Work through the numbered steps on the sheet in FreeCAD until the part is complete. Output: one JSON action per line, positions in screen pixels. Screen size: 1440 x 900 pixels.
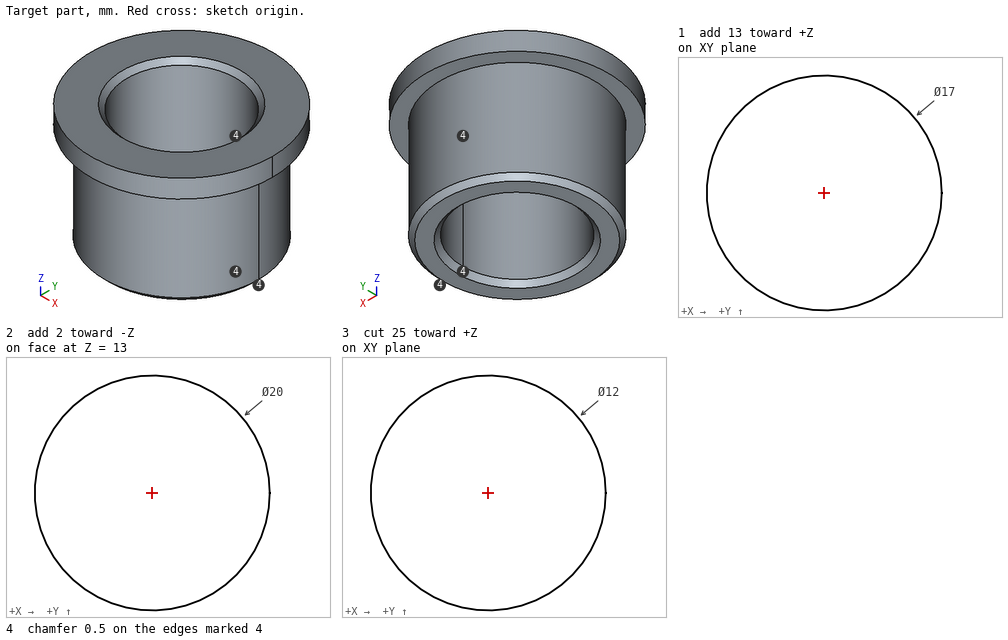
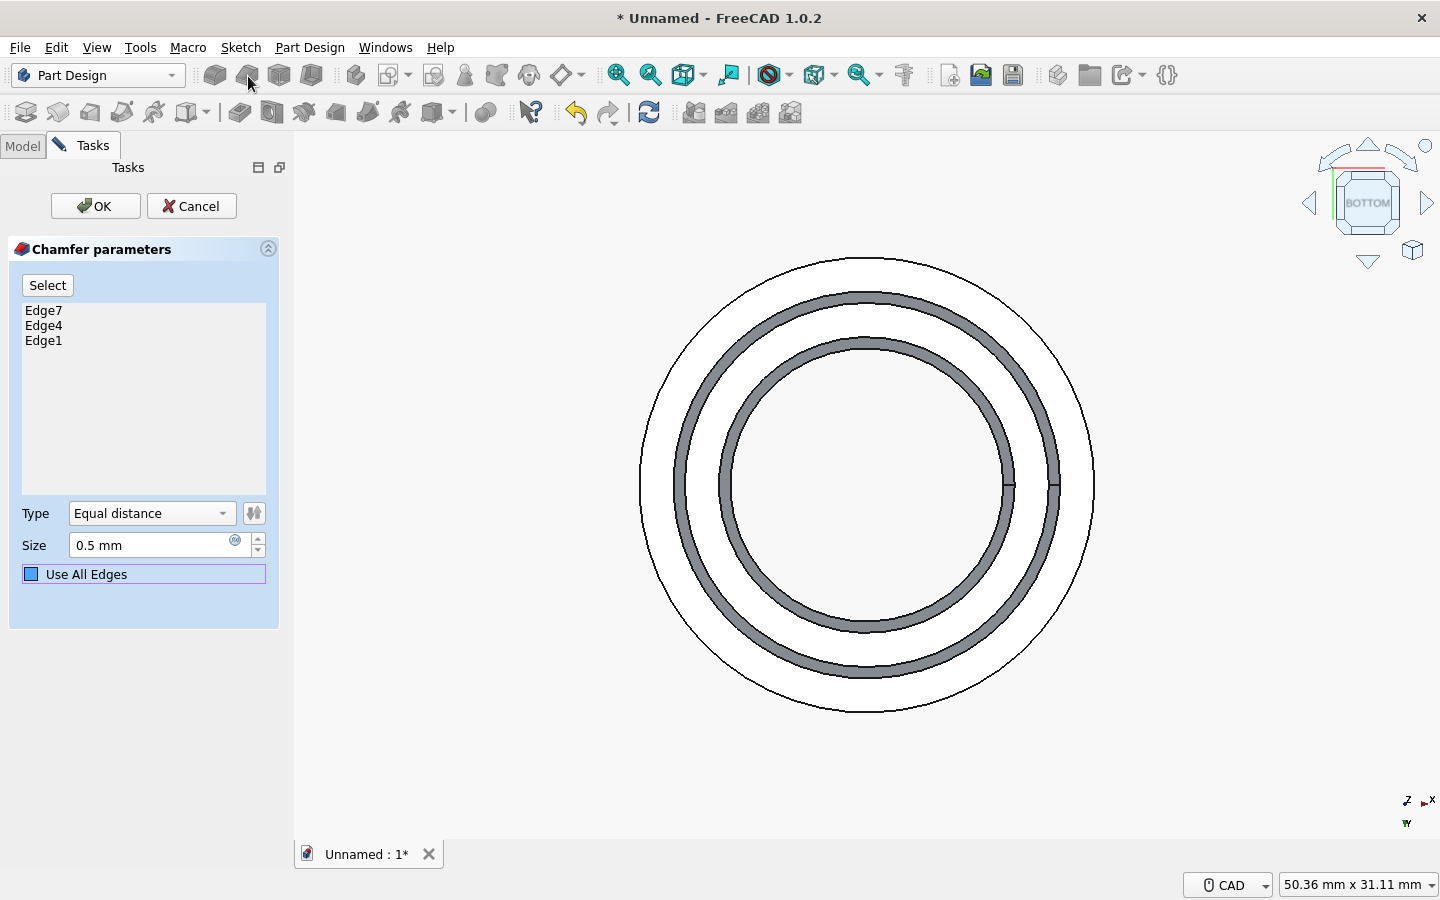
{"action": "left_click", "coordinate": [96, 206]}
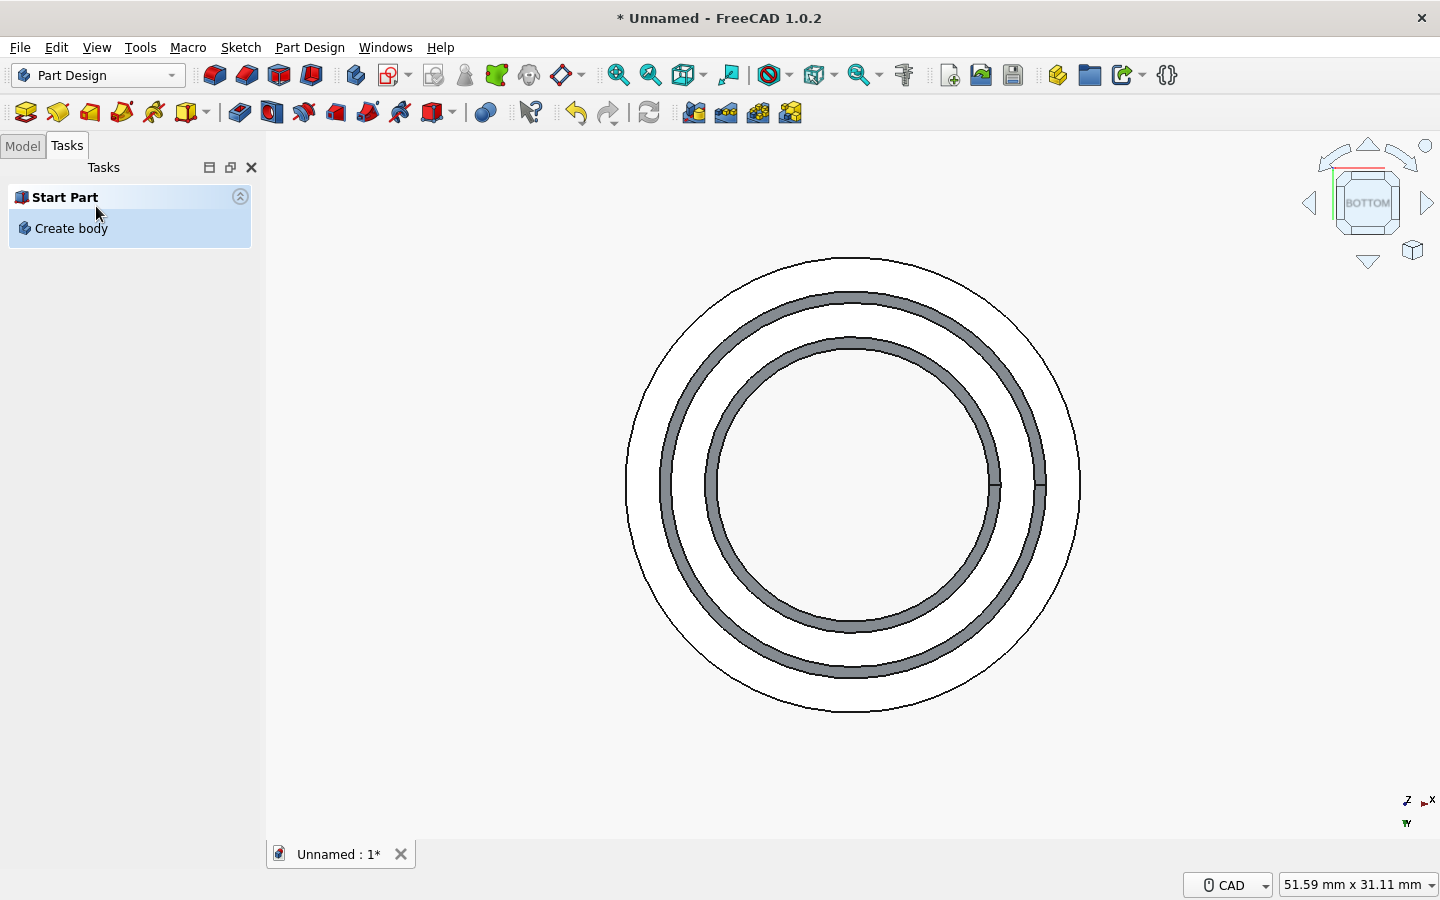
{"action": "key", "text": "0"}